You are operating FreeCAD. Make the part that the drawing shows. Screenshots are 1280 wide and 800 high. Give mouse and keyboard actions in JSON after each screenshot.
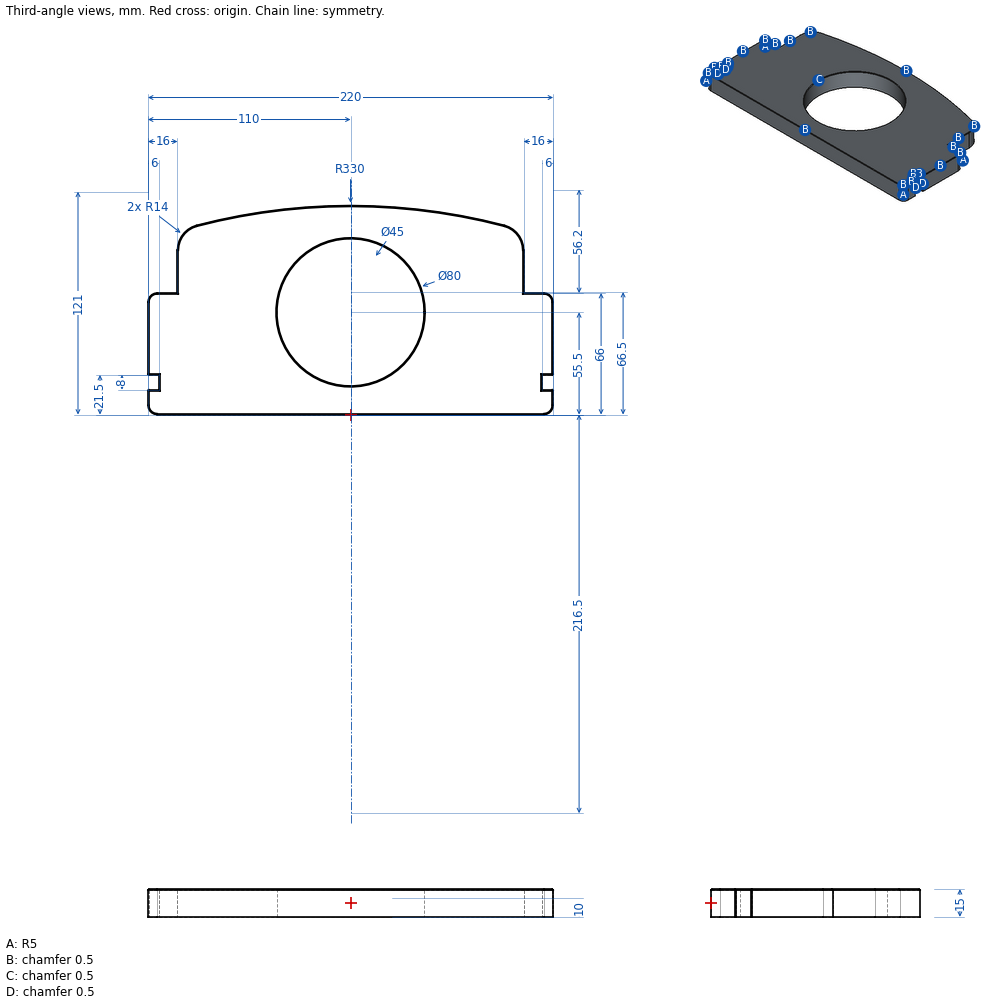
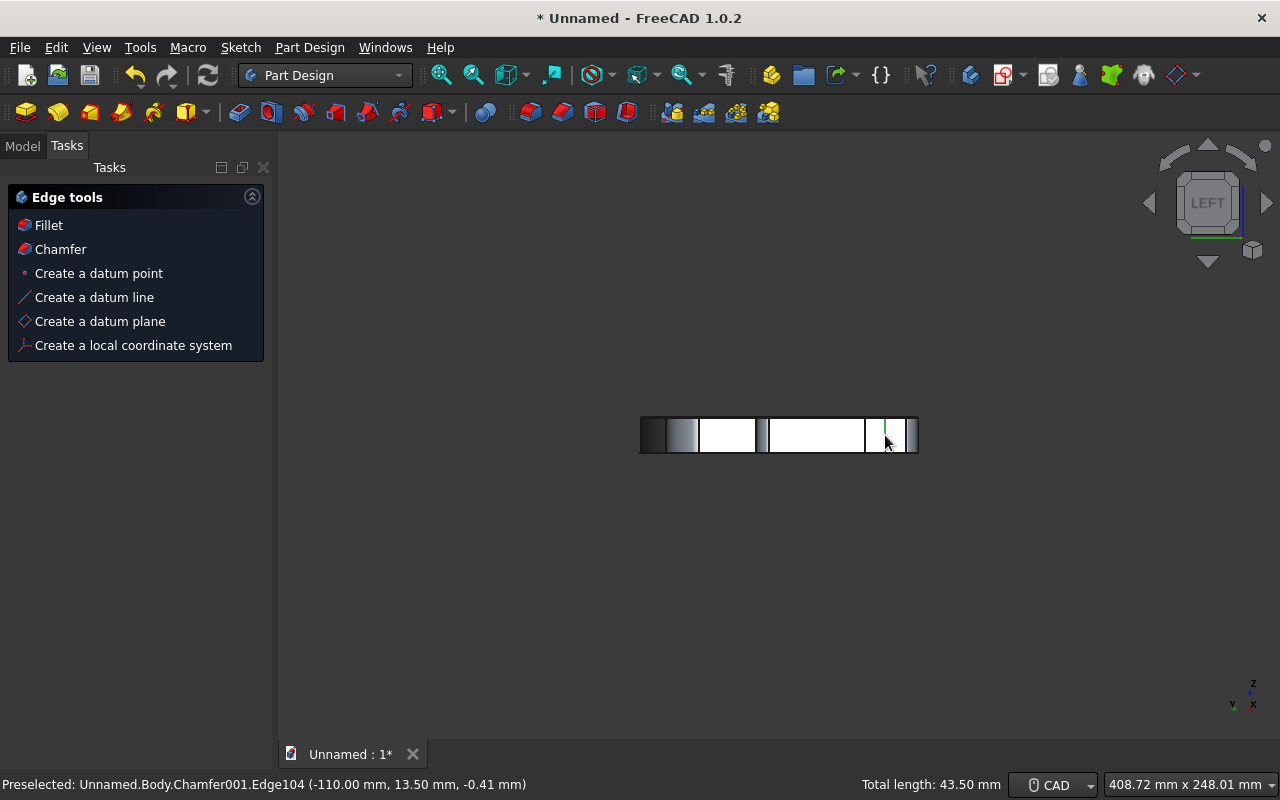
{"action": "left_click", "coordinate": [865, 435], "text": "ctrl"}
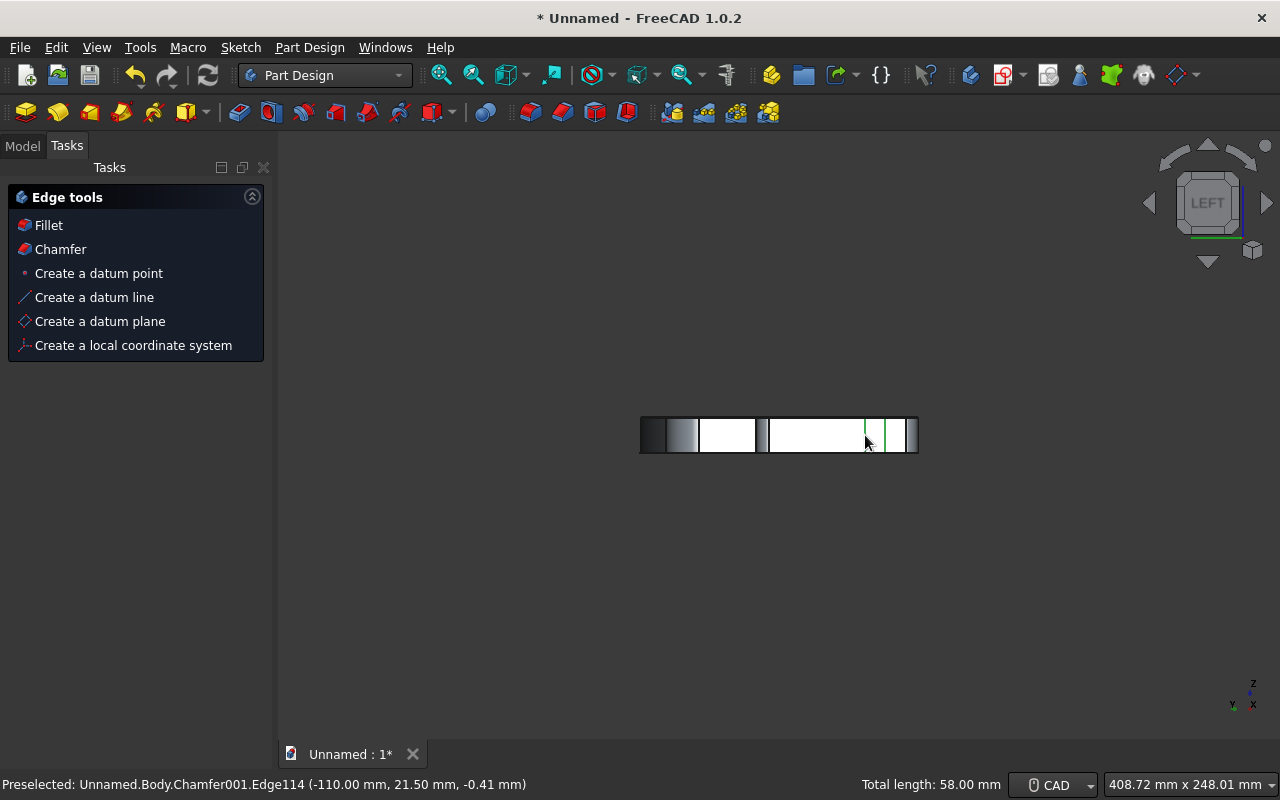
{"action": "left_click", "coordinate": [564, 112]}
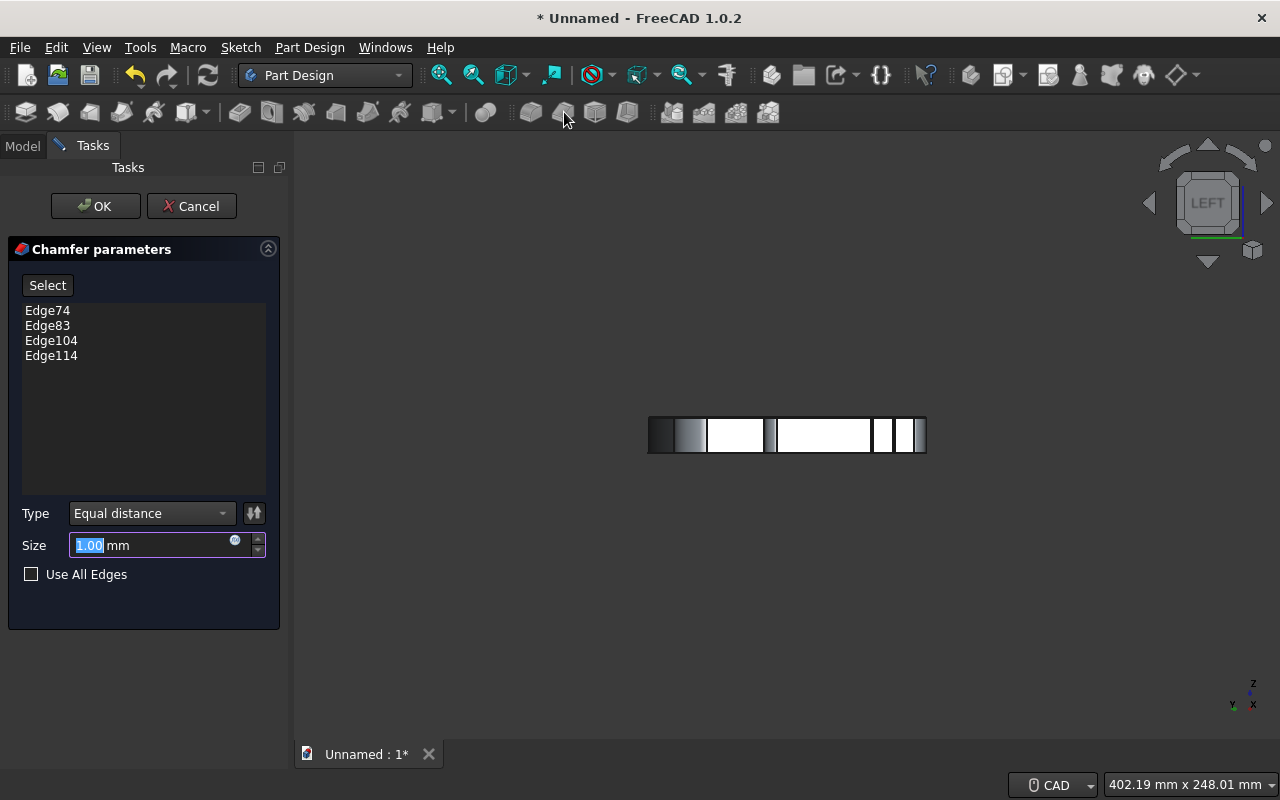
{"action": "type", "text": "0.5"}
{"action": "key", "text": "Tab"}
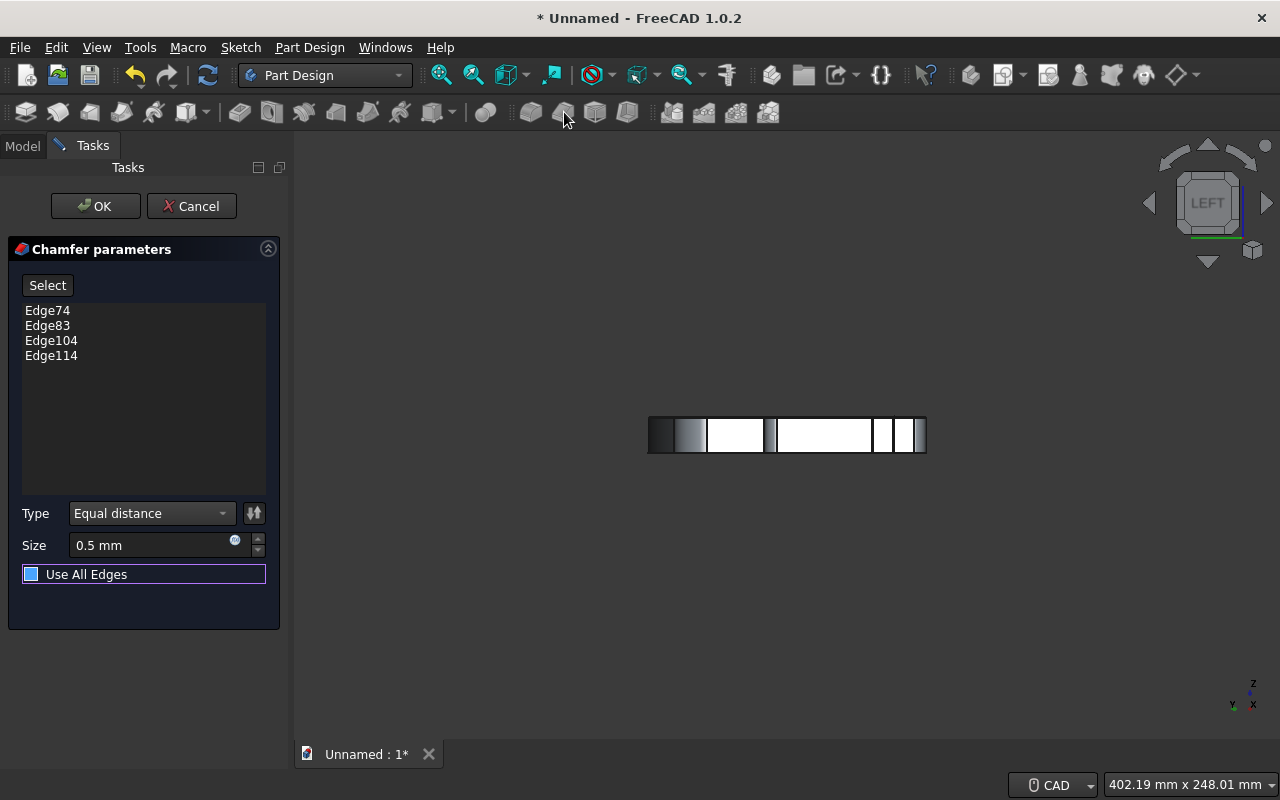
{"action": "left_click", "coordinate": [96, 206]}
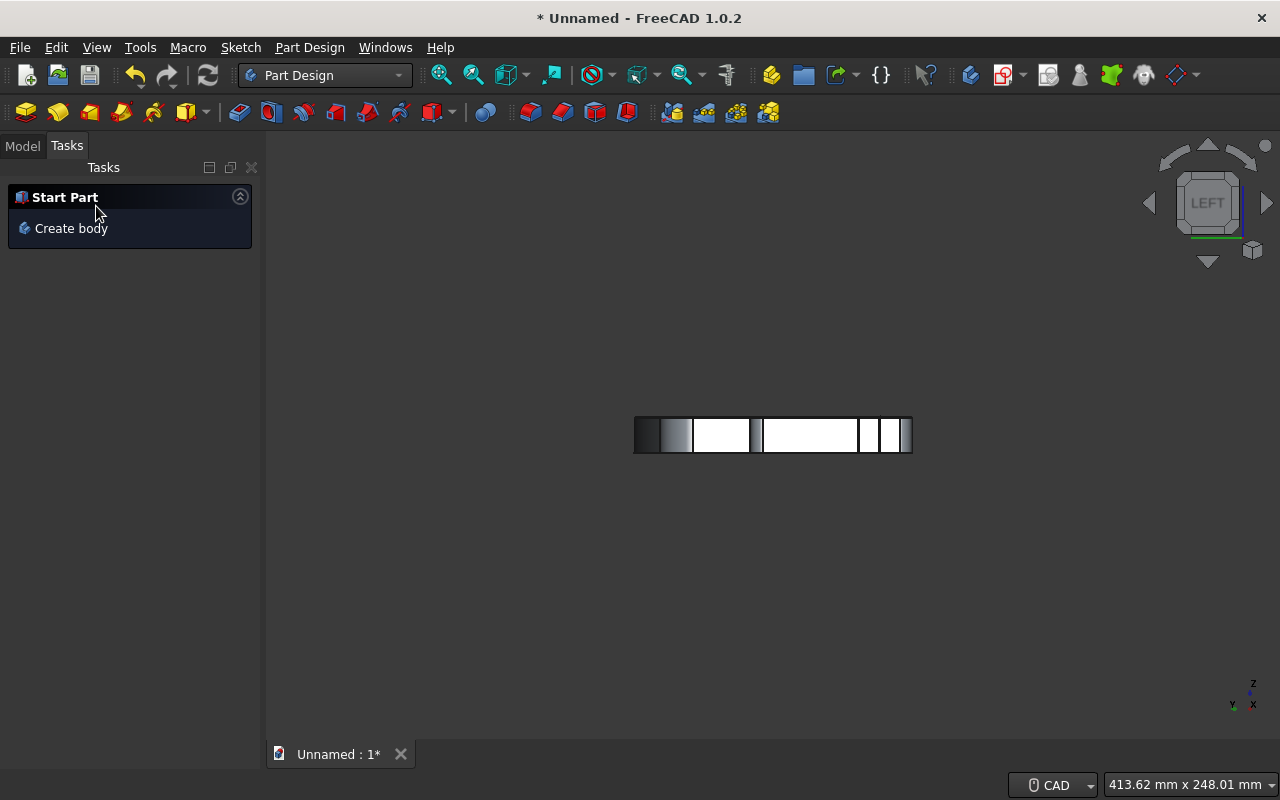
{"action": "key", "text": "0"}